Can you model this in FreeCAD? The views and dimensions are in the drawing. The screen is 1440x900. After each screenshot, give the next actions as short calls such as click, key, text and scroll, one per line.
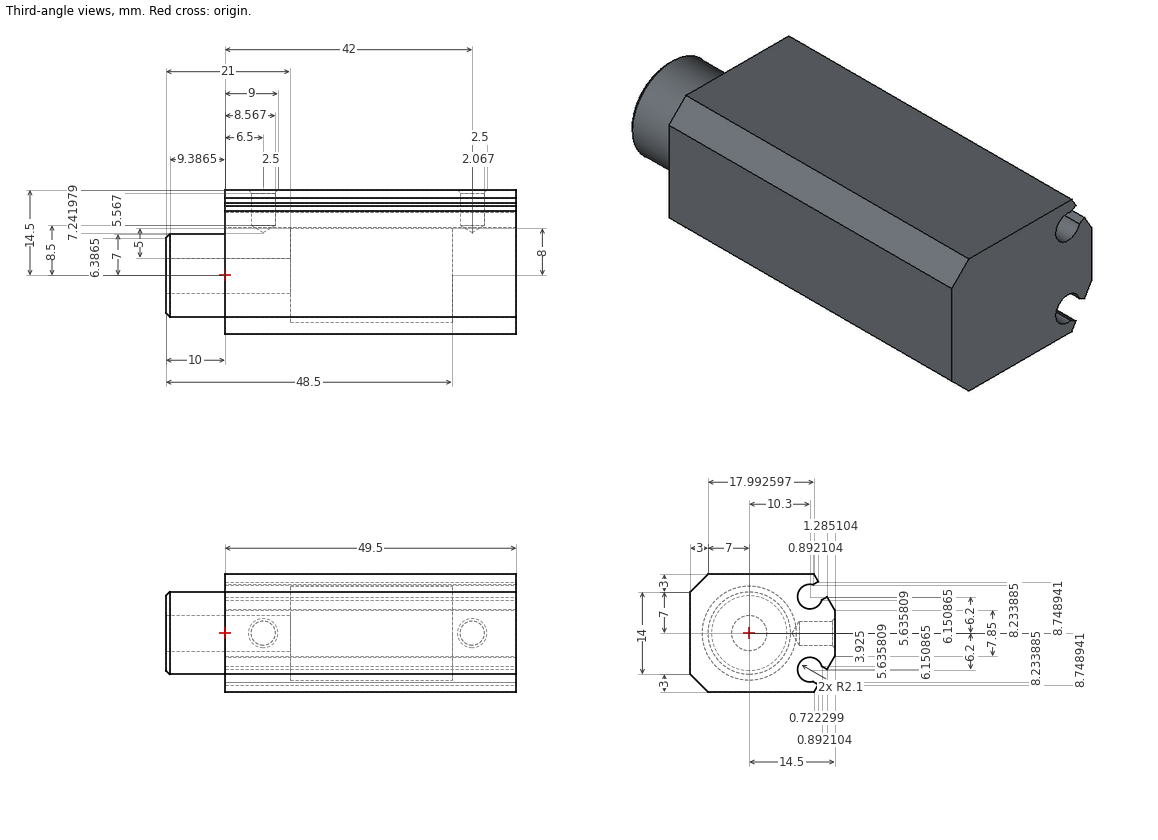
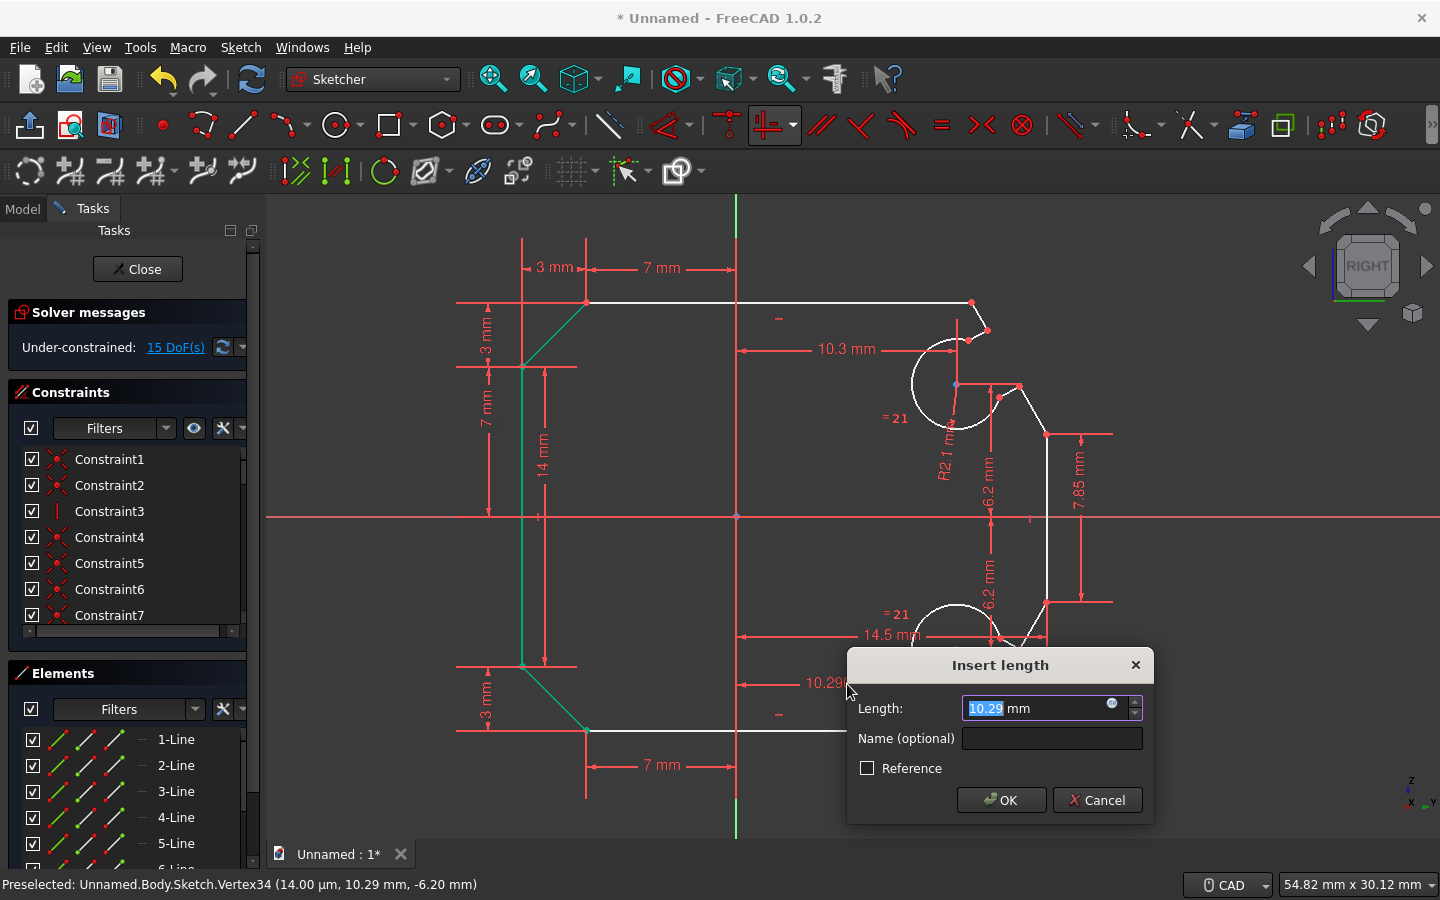
text(10.3)
key(Return)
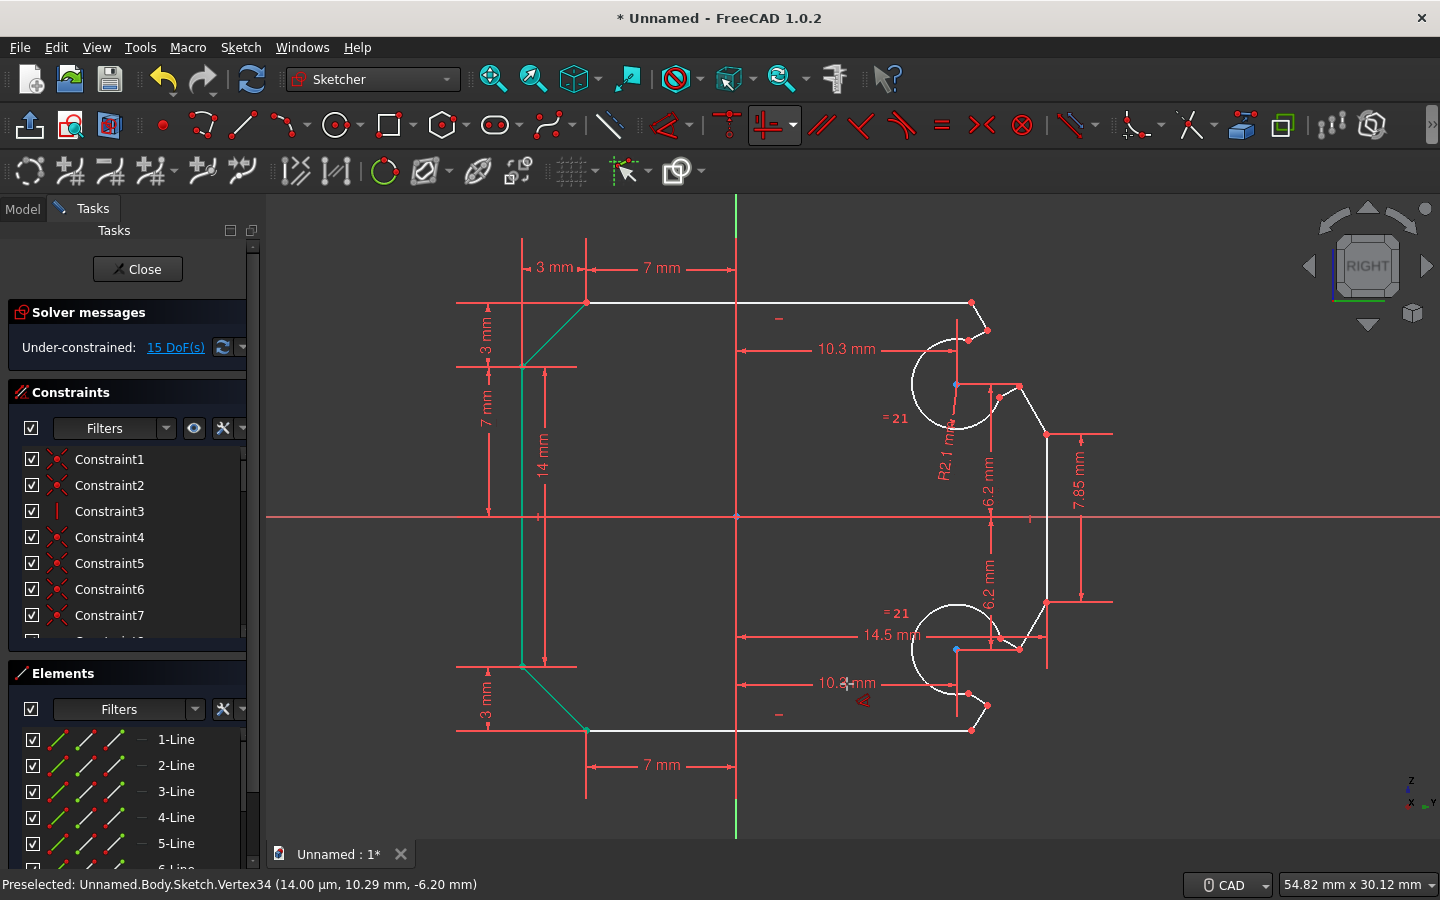
click(1047, 602)
click(1081, 560)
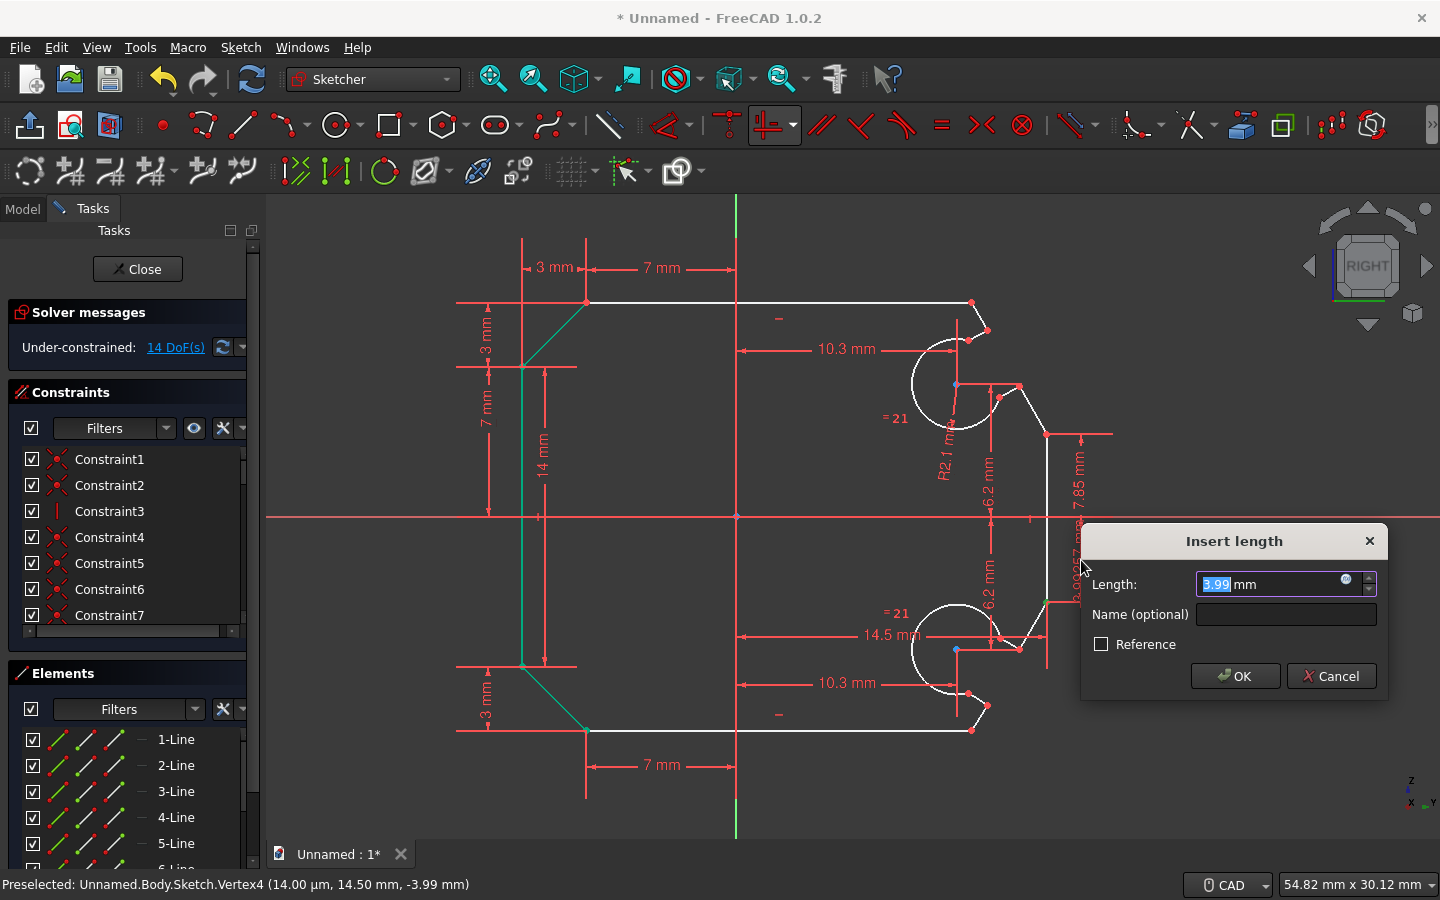
text(3.925)
key(Return)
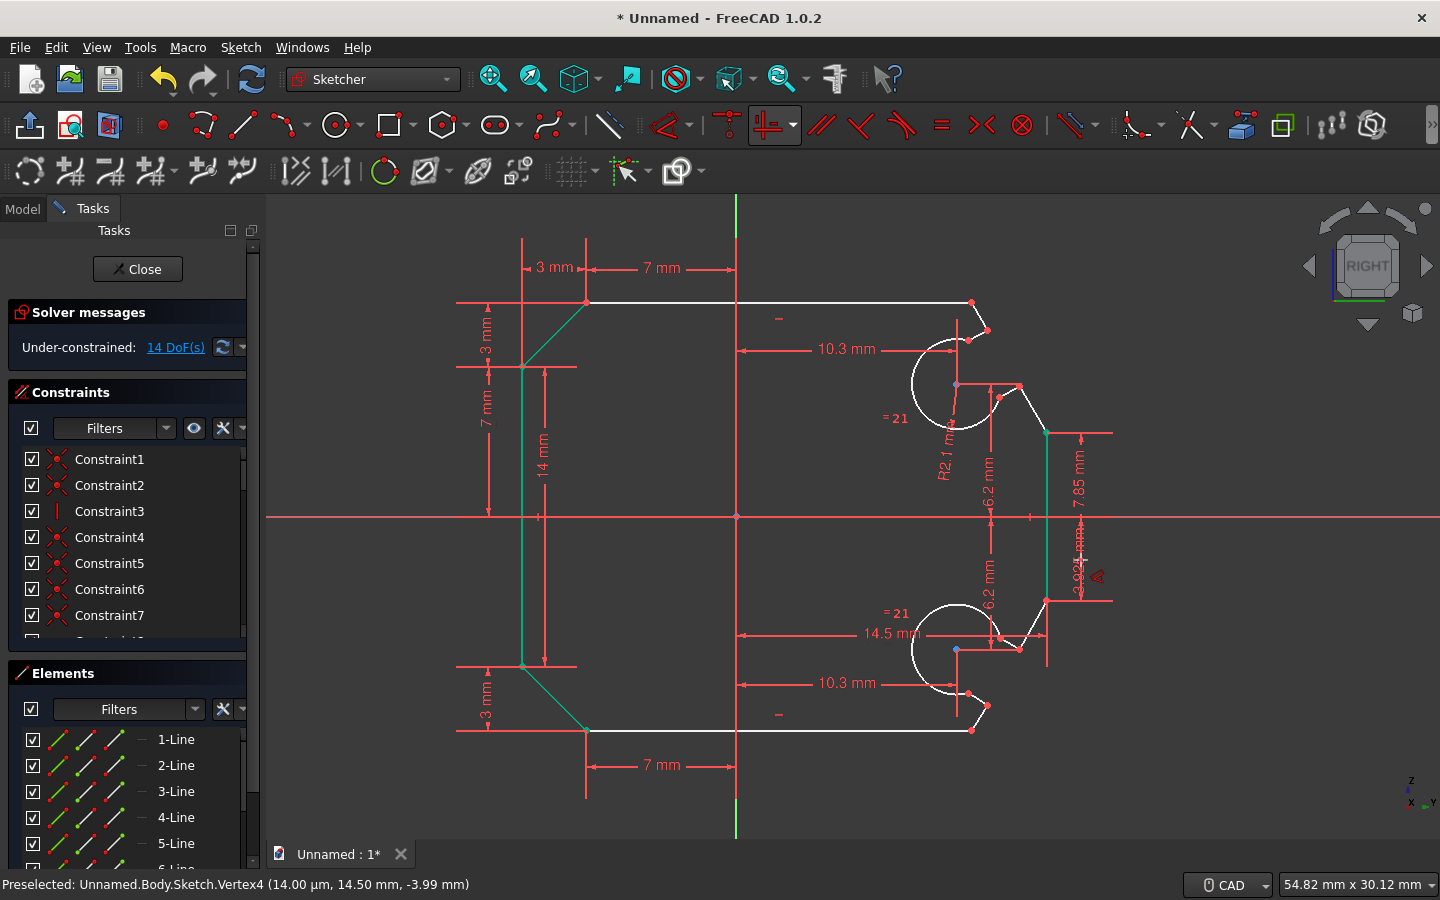
click(856, 303)
click(779, 269)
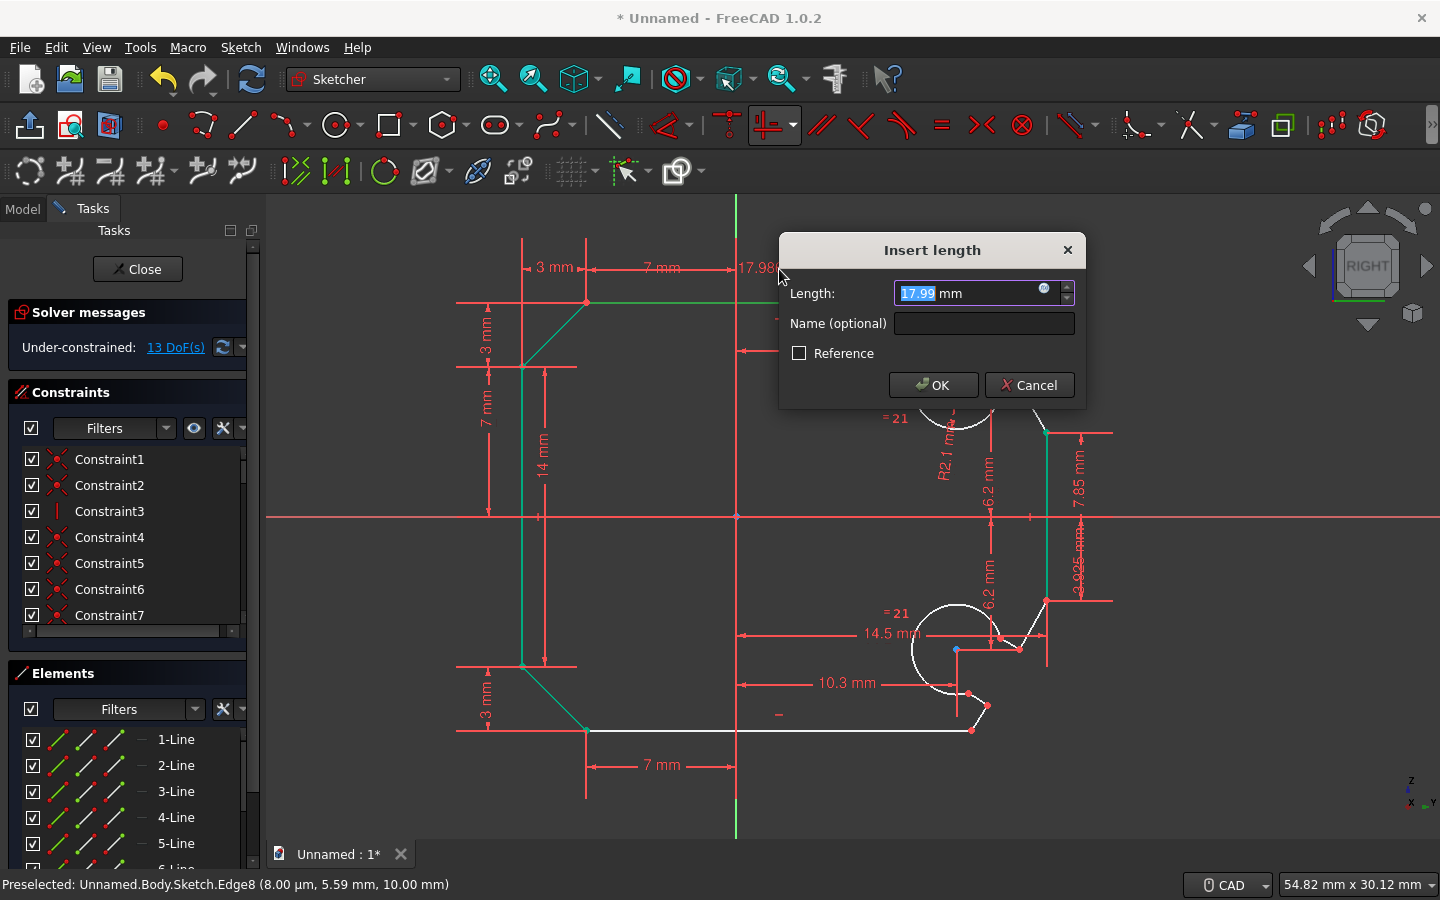
text(17.992597)
key(Return)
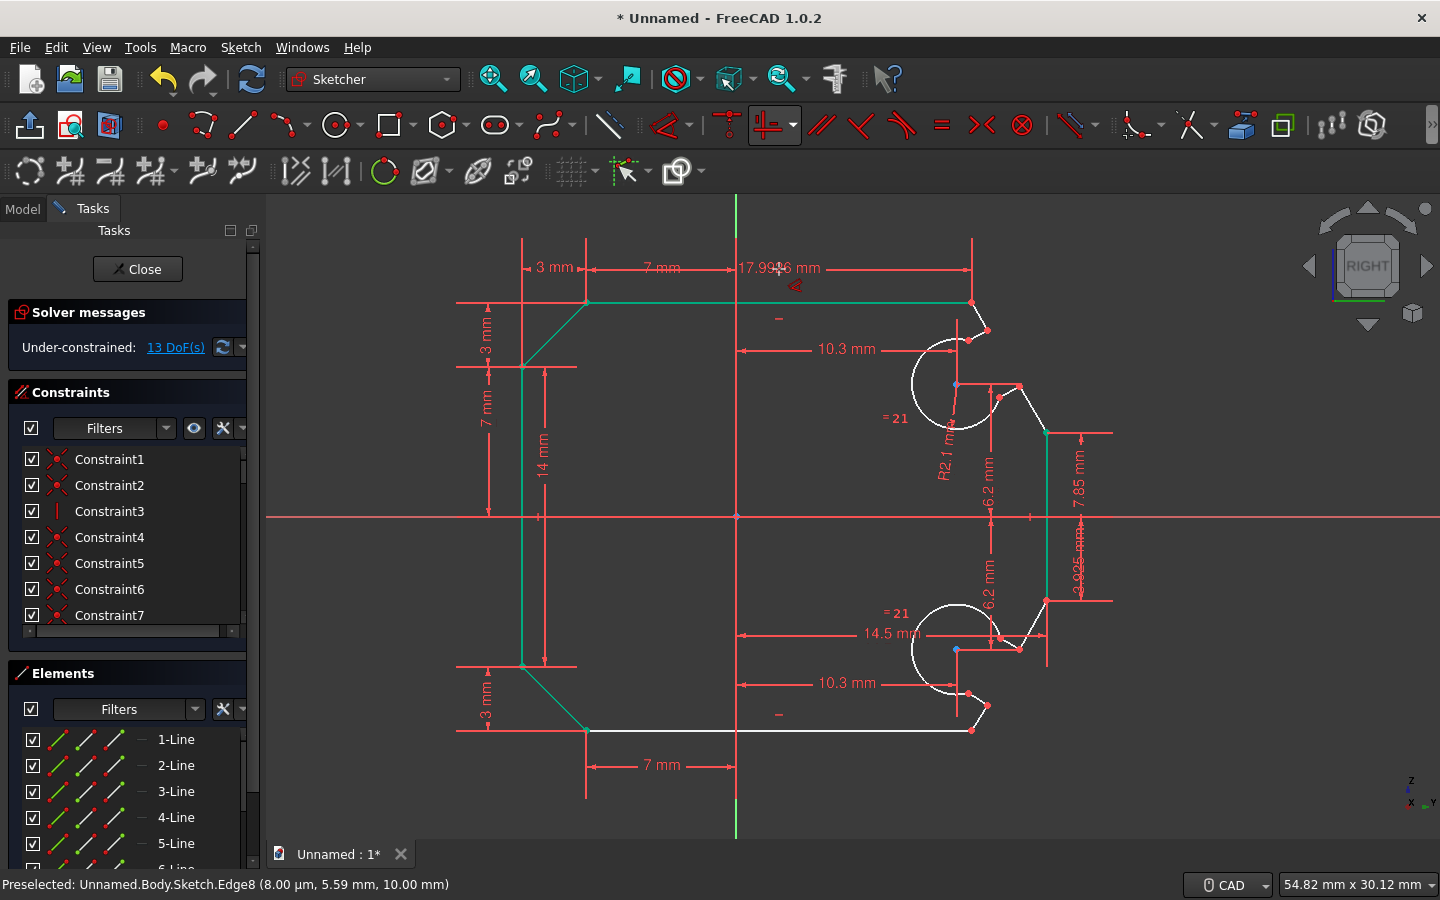
click(702, 731)
click(779, 765)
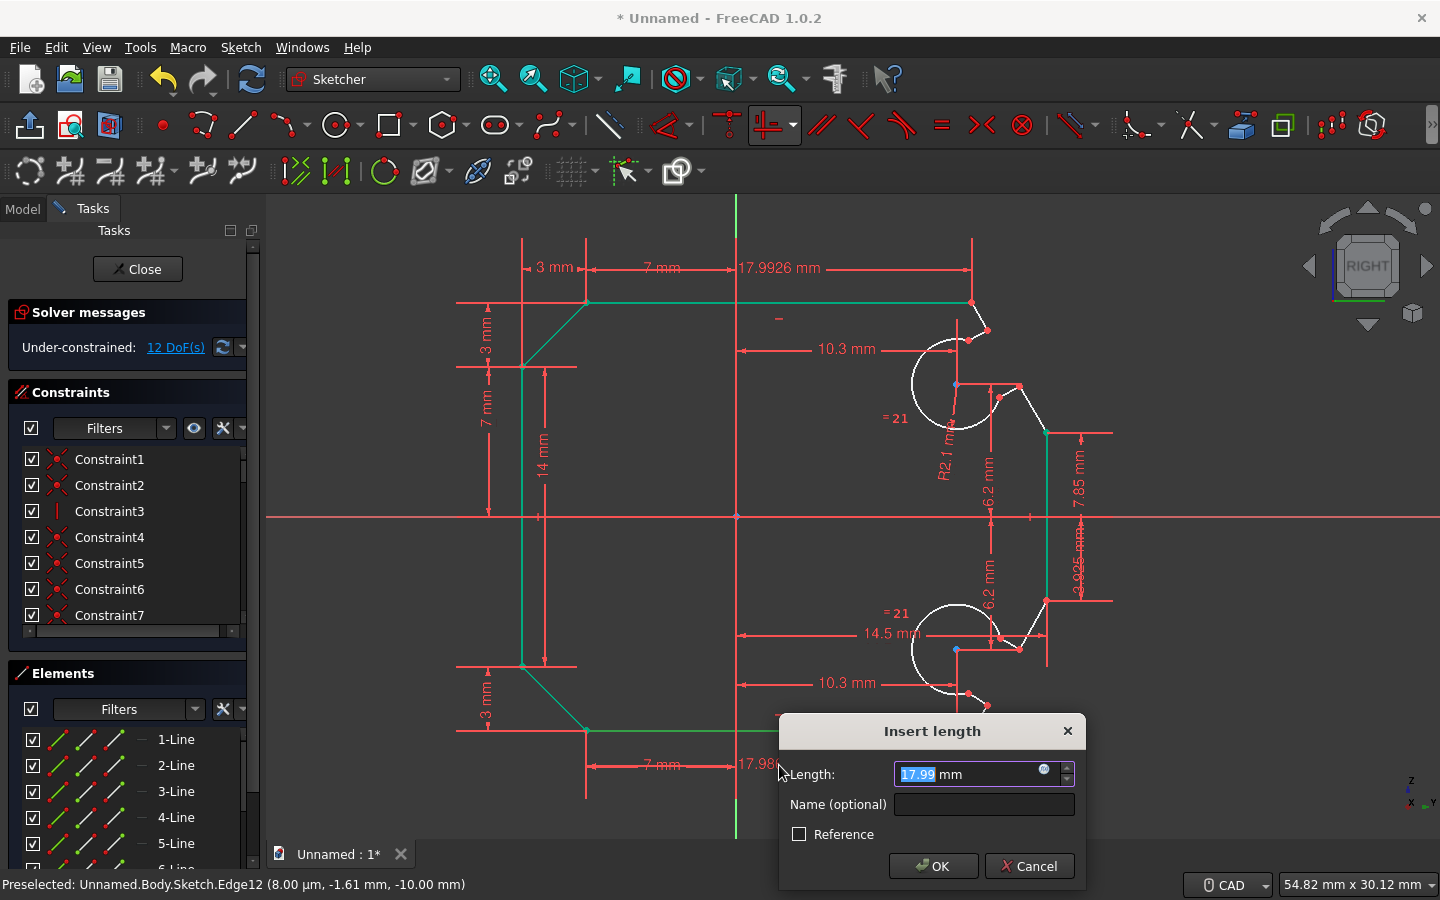
text(17.992597)
key(Return)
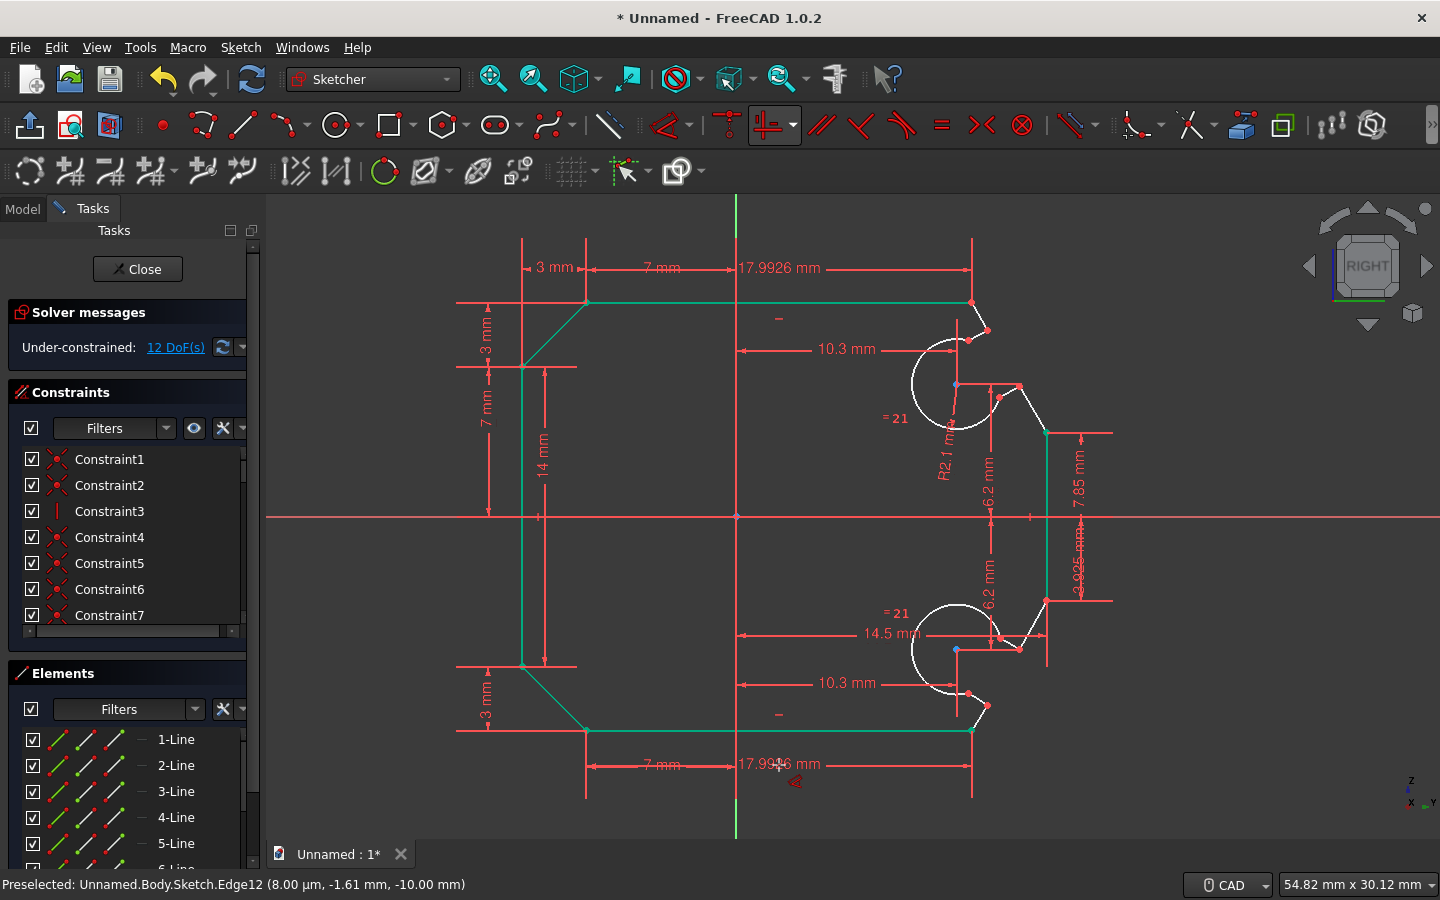
click(1001, 638)
click(702, 578)